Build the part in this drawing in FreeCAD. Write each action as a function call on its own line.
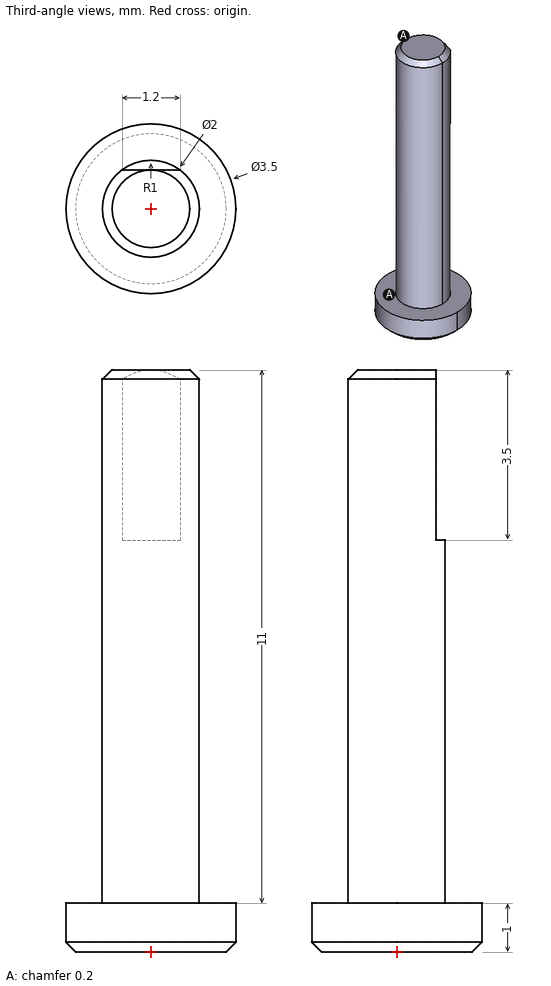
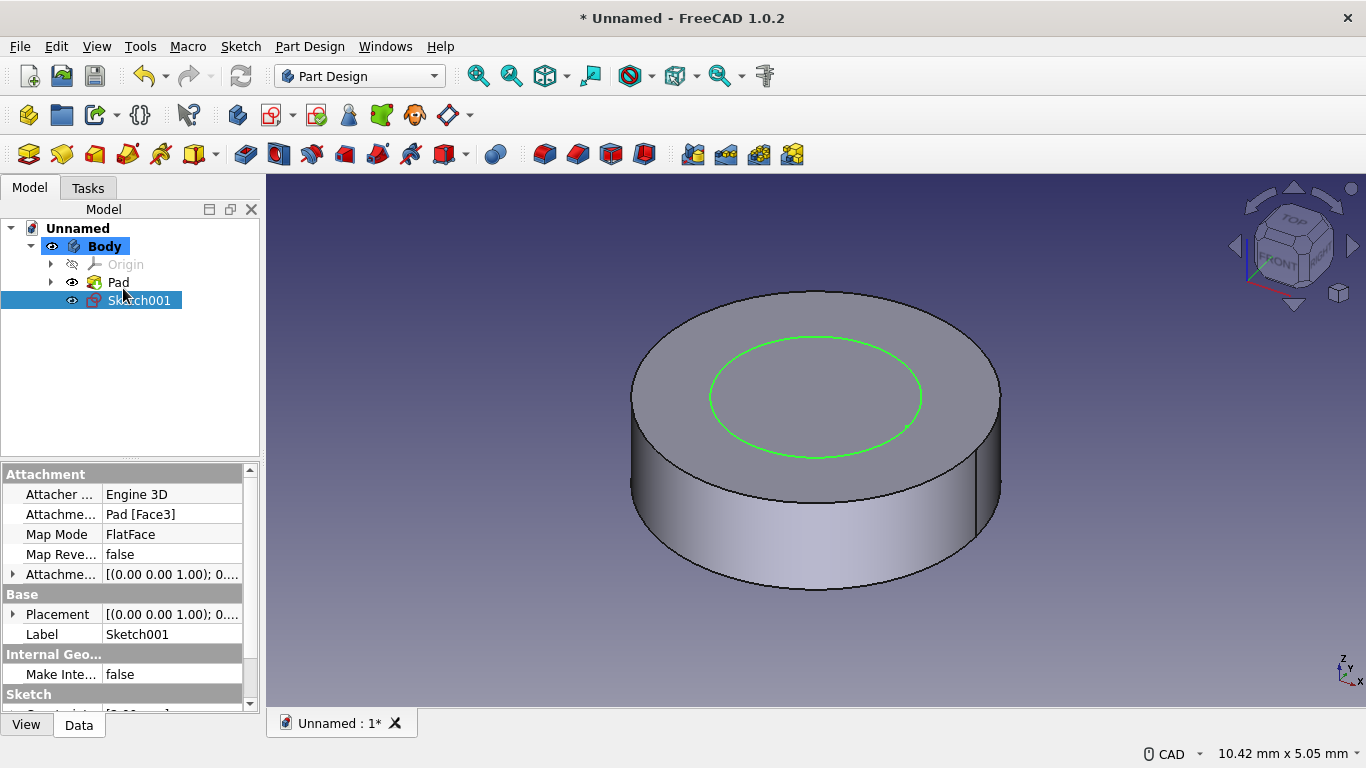
click(29, 154)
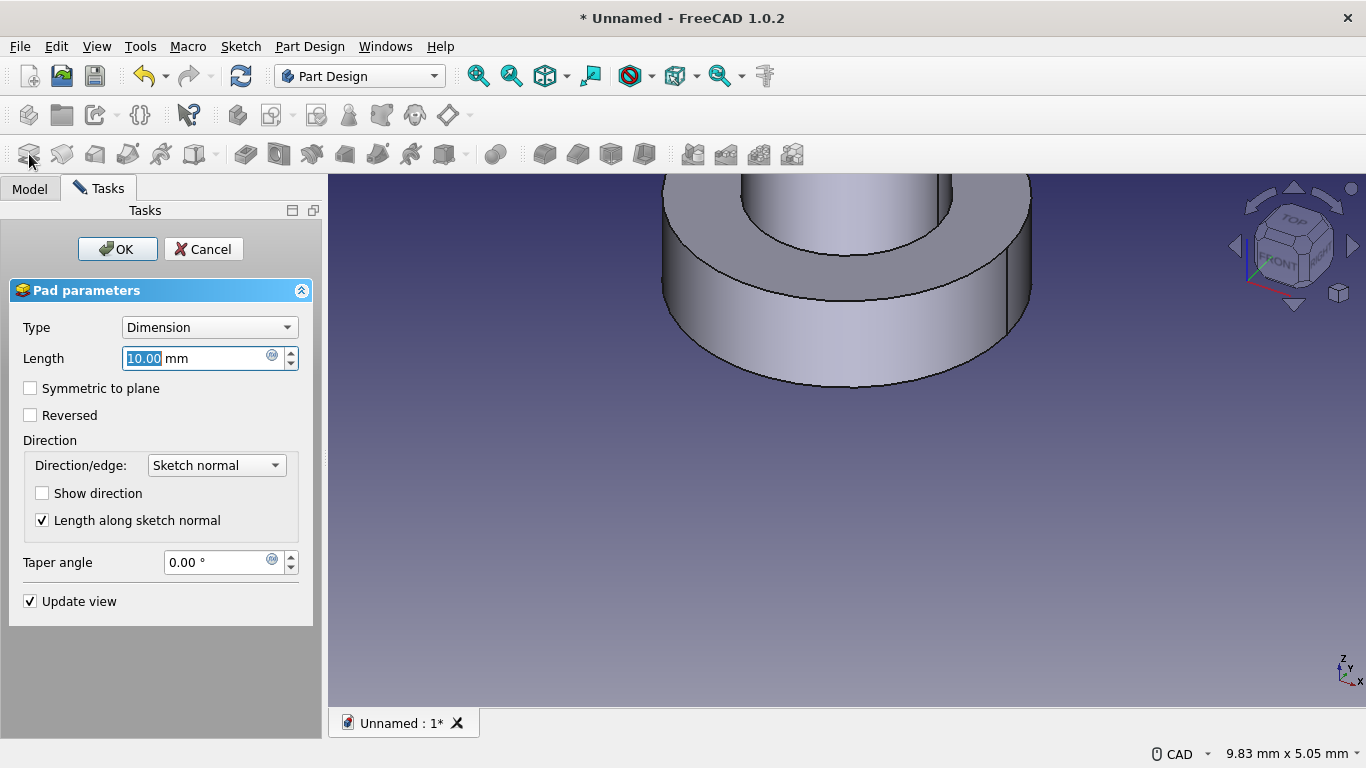
text(11)
key(Tab)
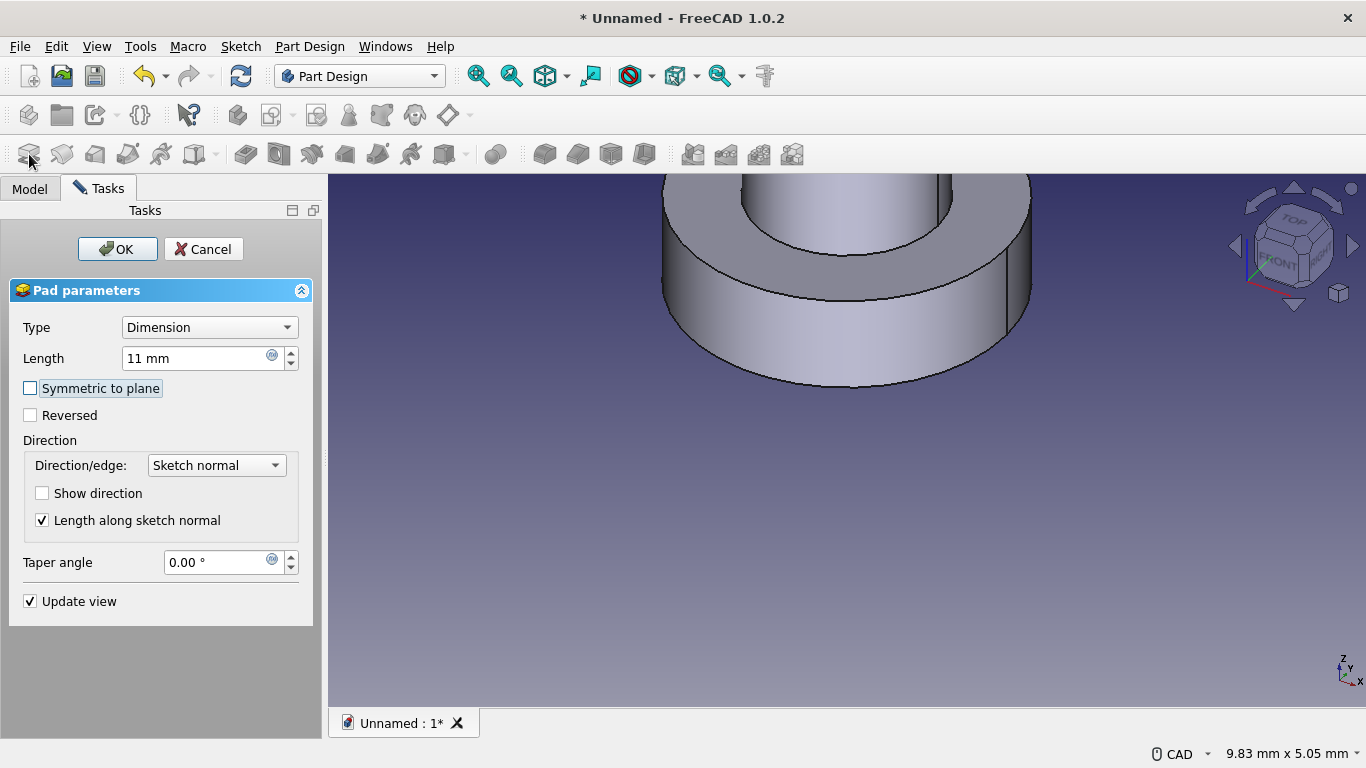
click(118, 249)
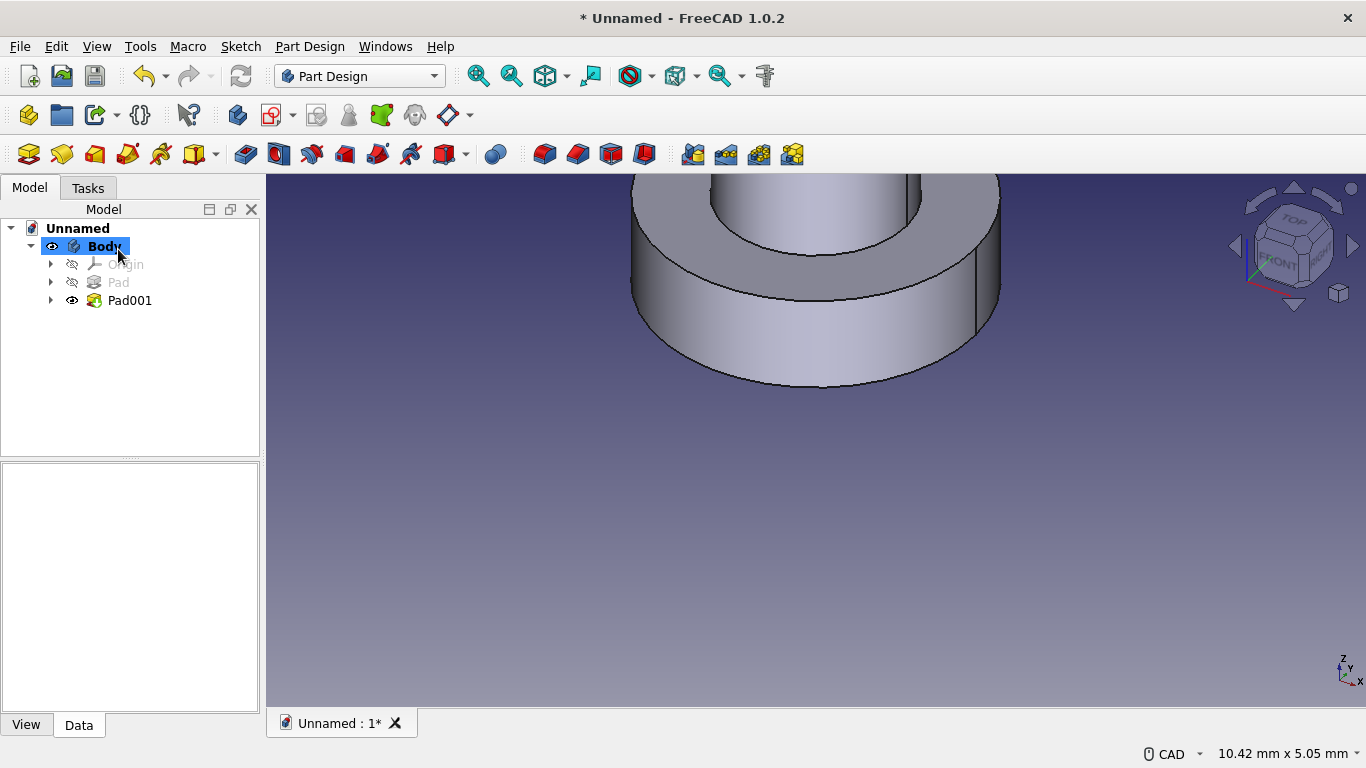
key(v)
key(f)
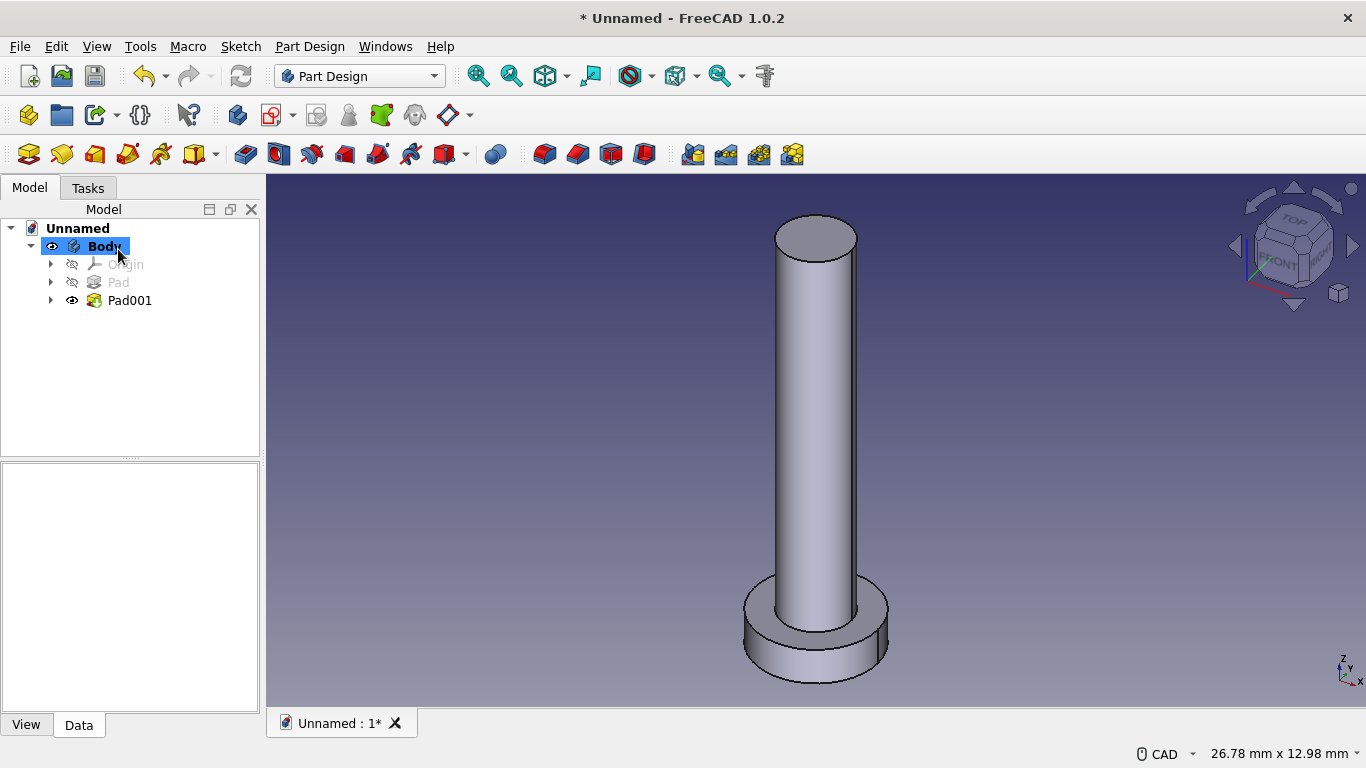
click(775, 240)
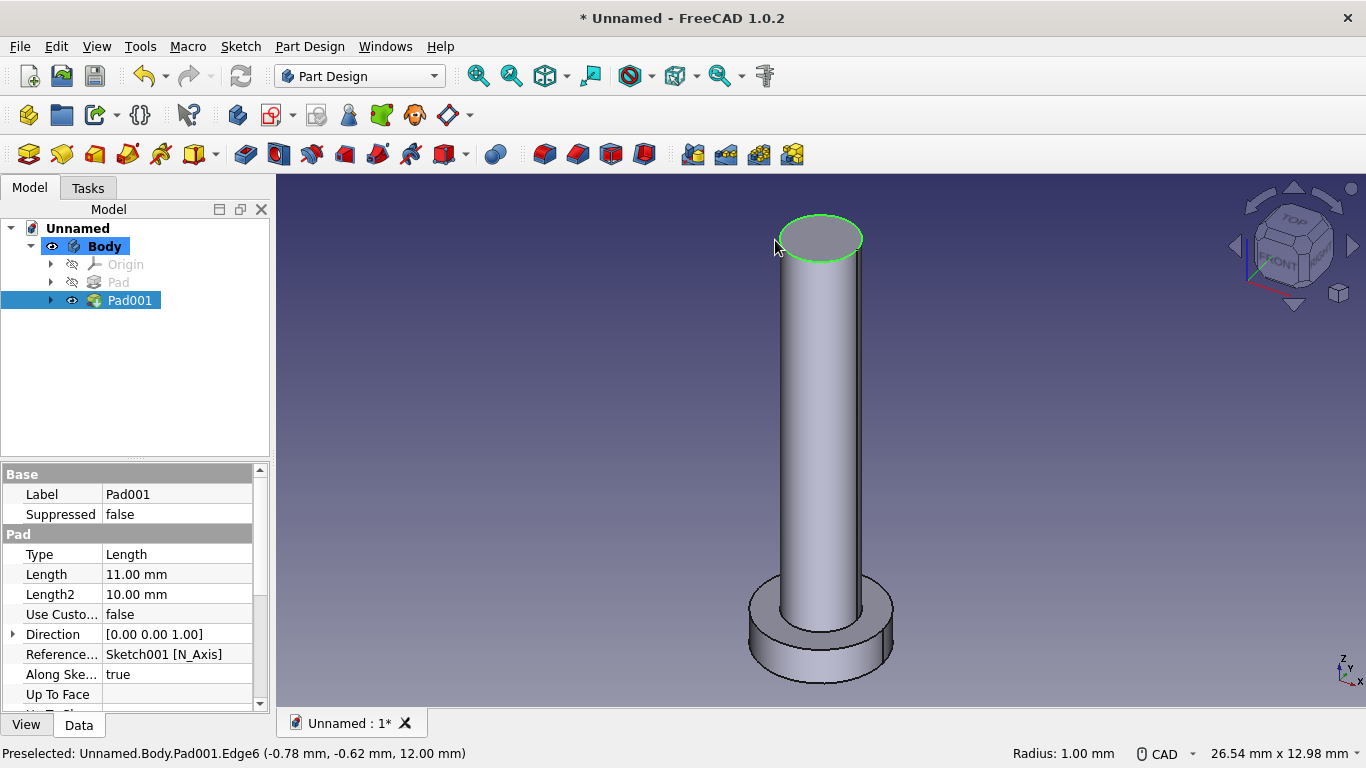
key(0)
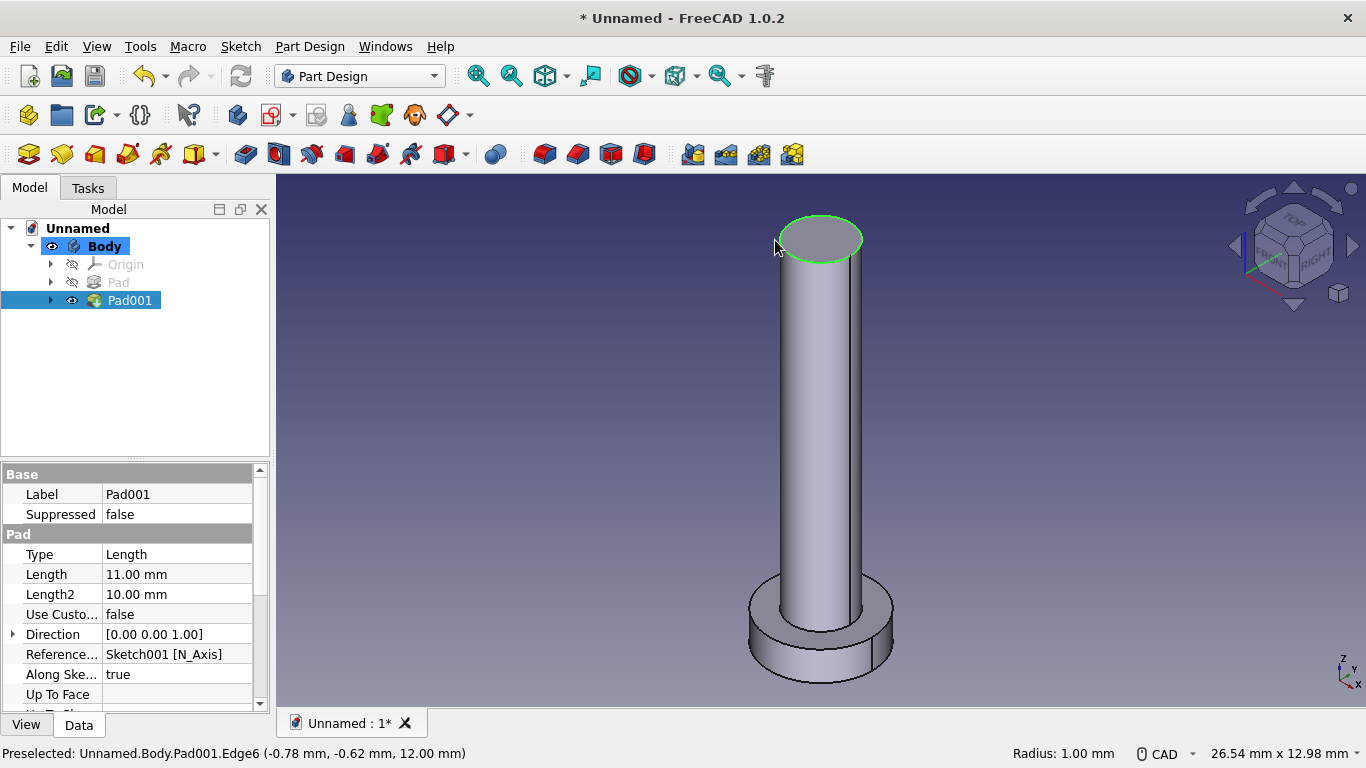
click(757, 660, ctrl)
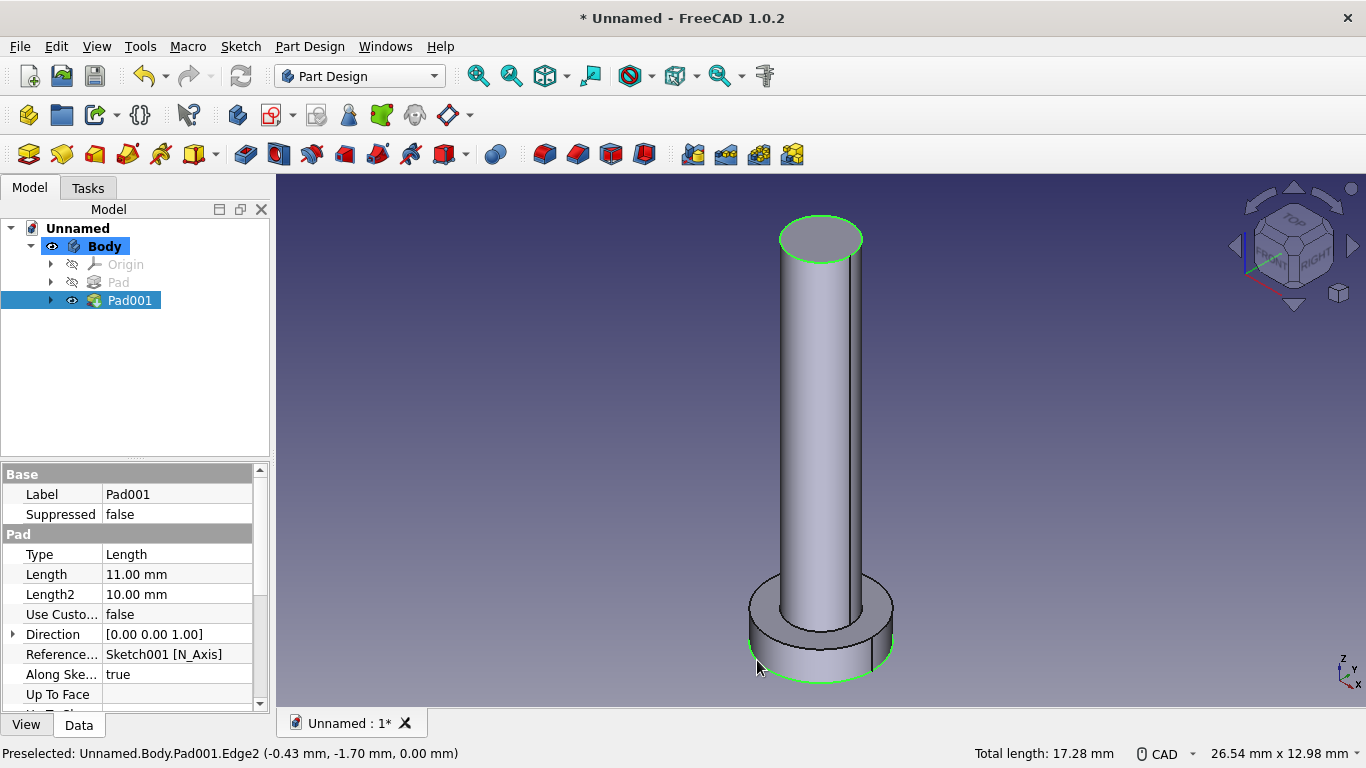
click(578, 154)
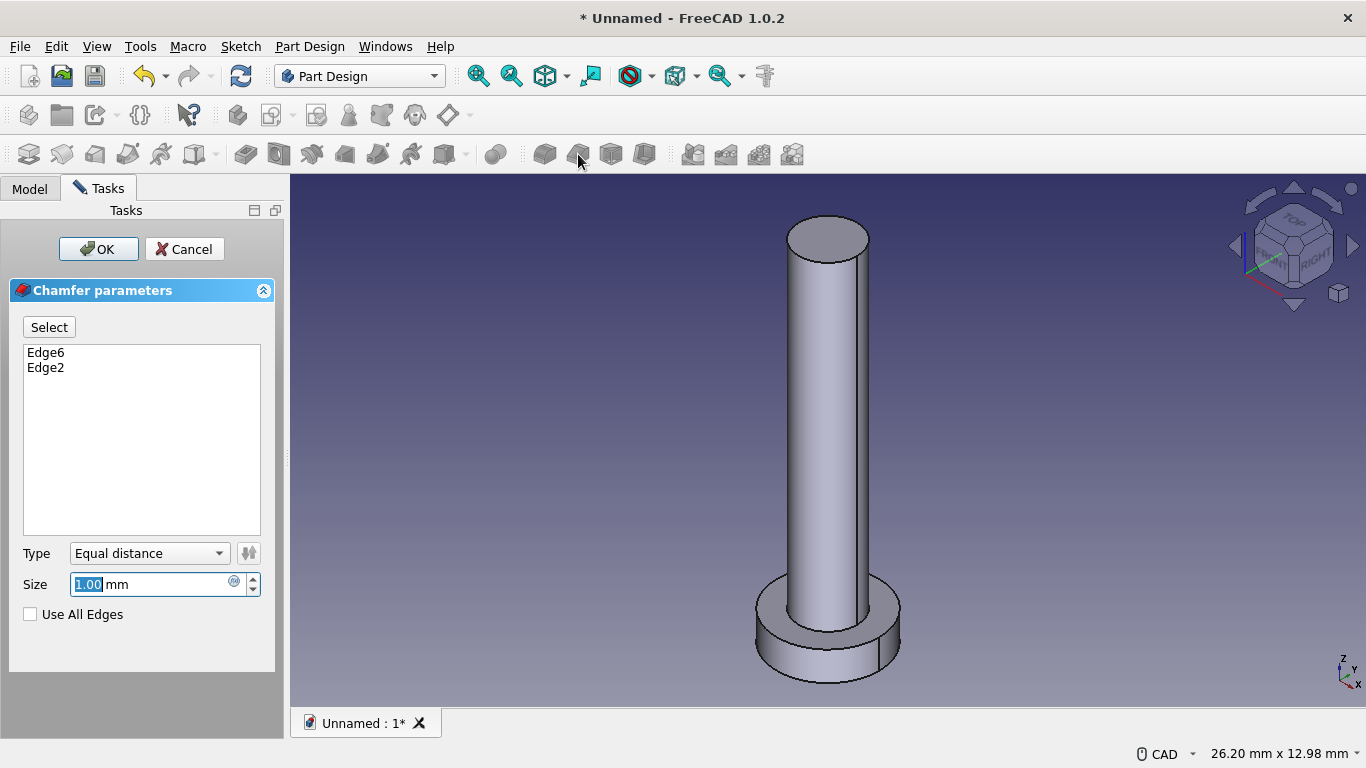
text(0.2)
key(Tab)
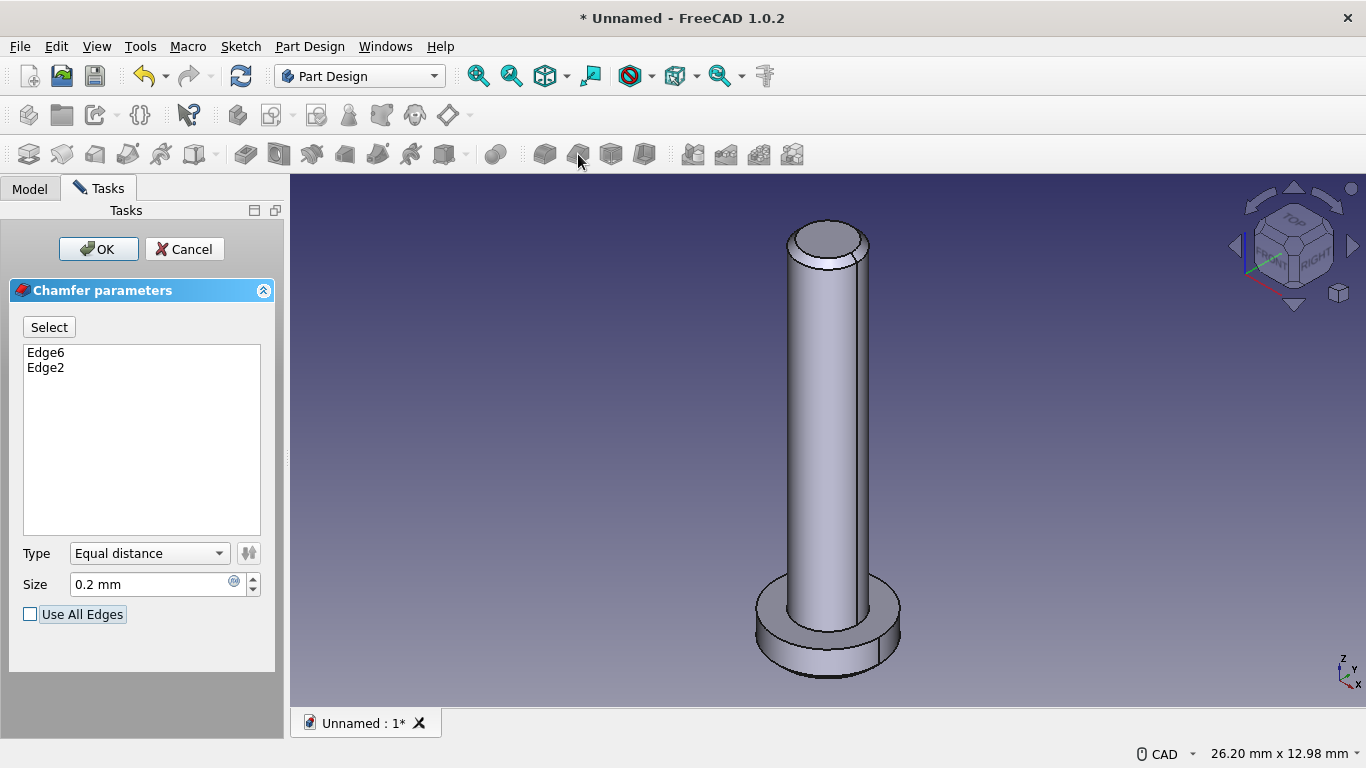
click(99, 249)